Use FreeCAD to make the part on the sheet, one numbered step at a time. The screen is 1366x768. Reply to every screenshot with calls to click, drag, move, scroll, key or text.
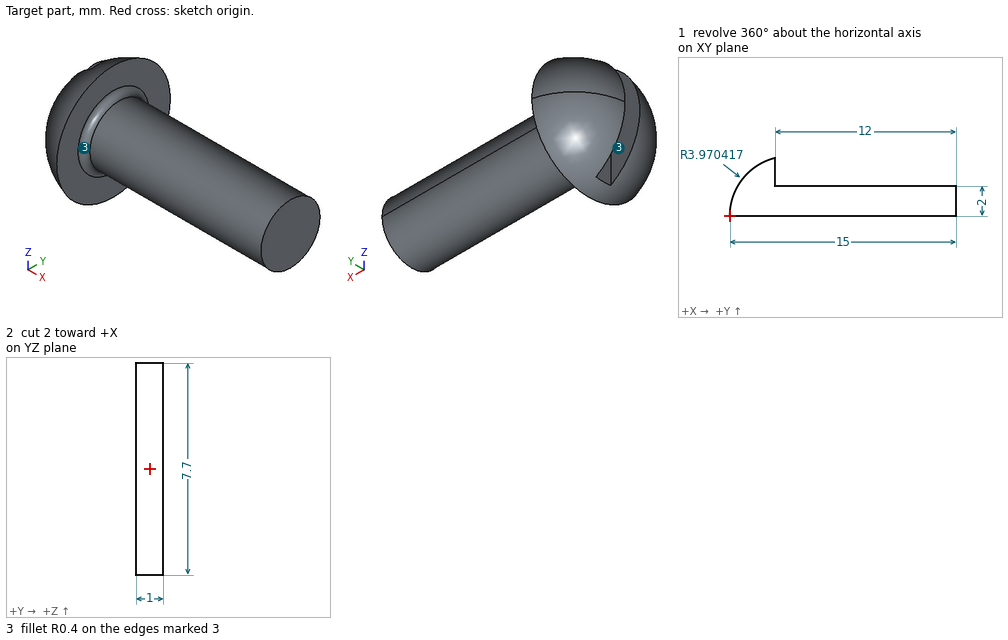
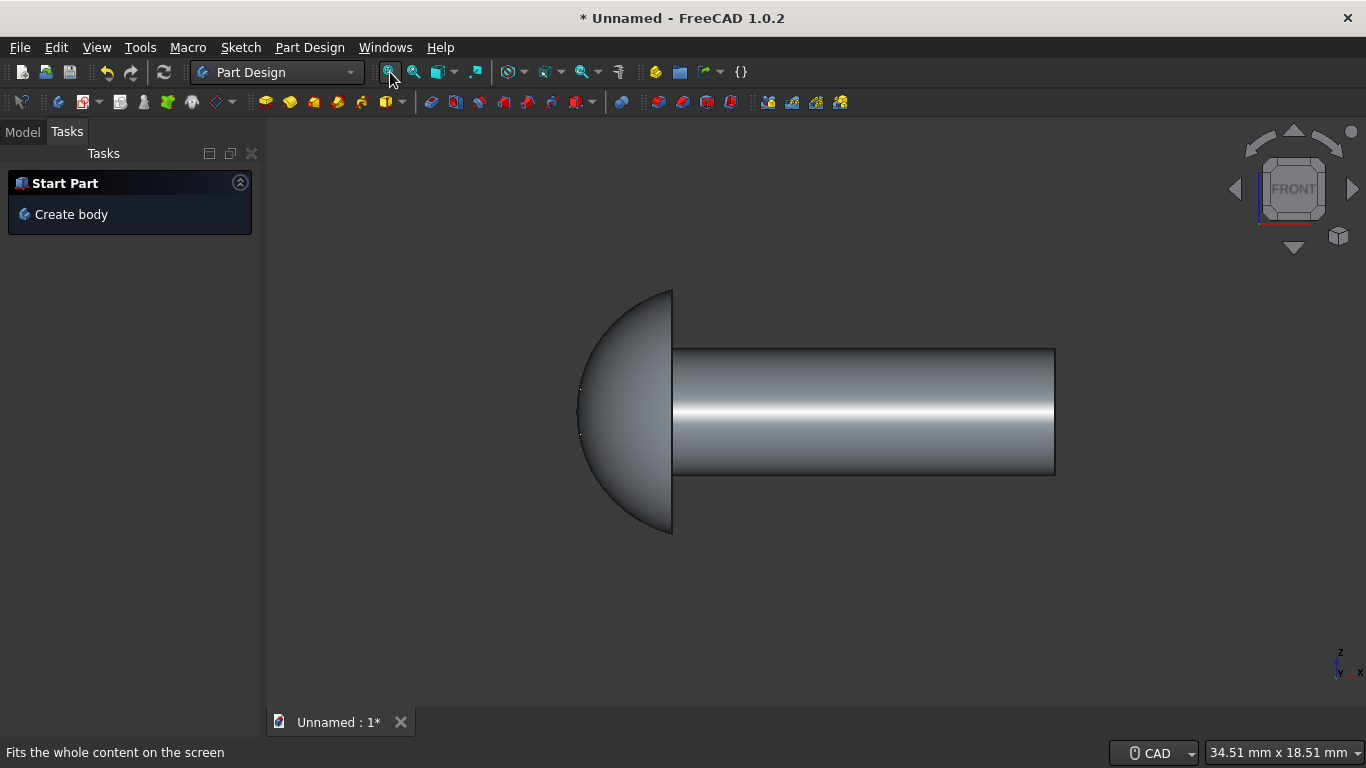
key(v)
key(f)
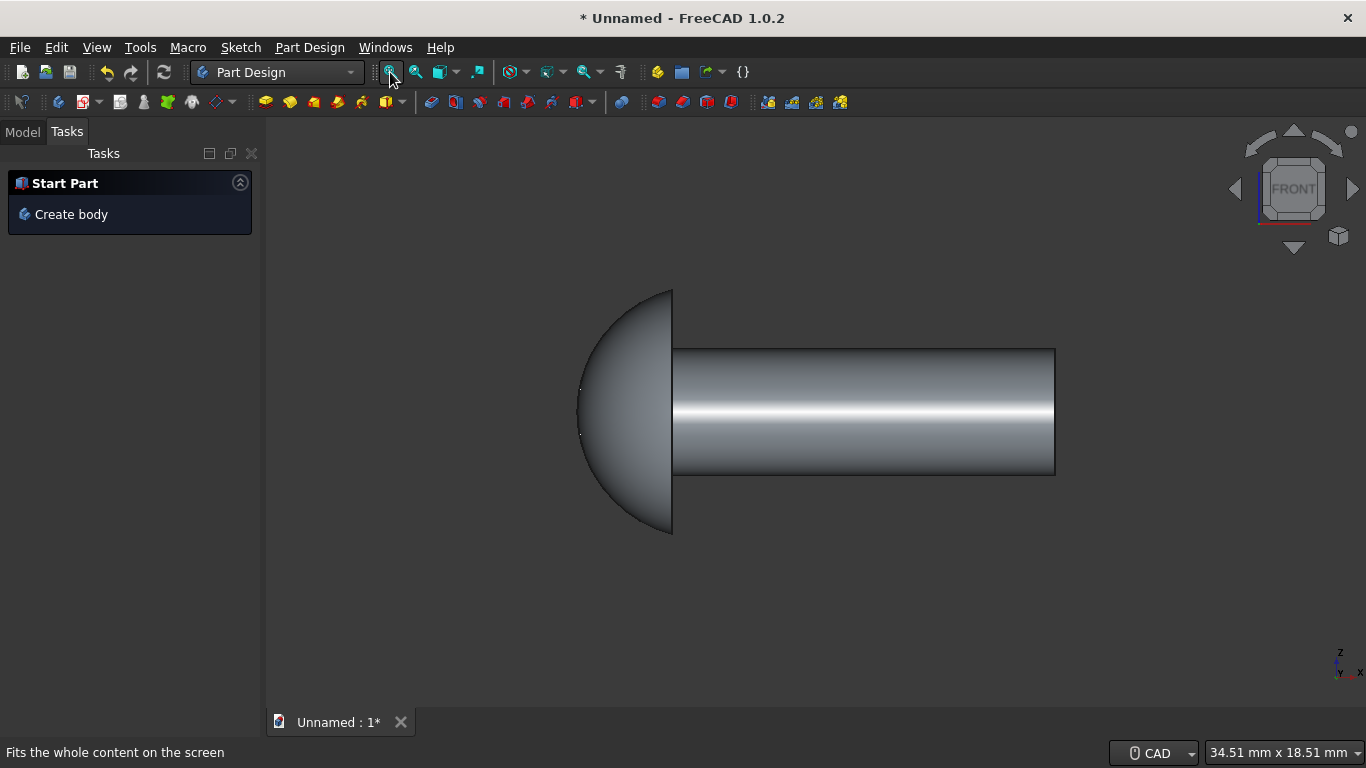
key(3)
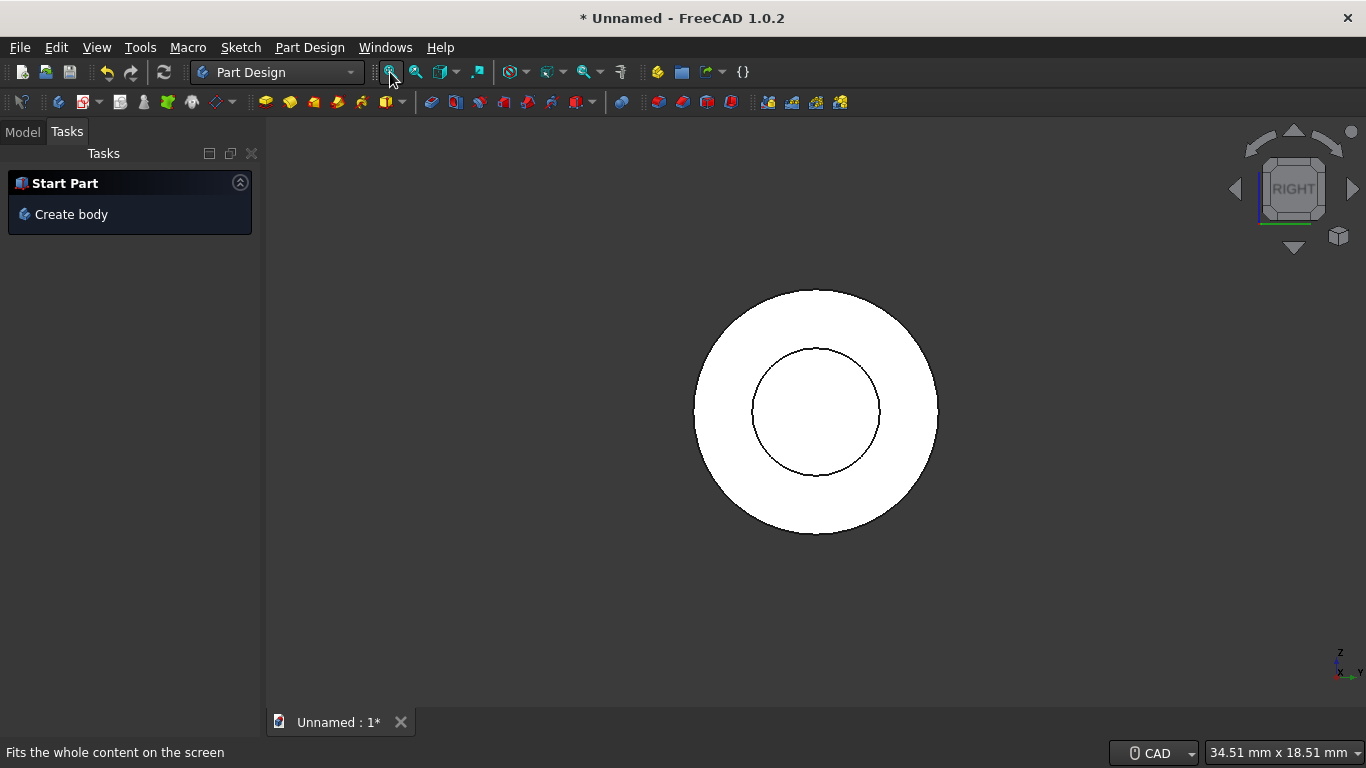
click(392, 72)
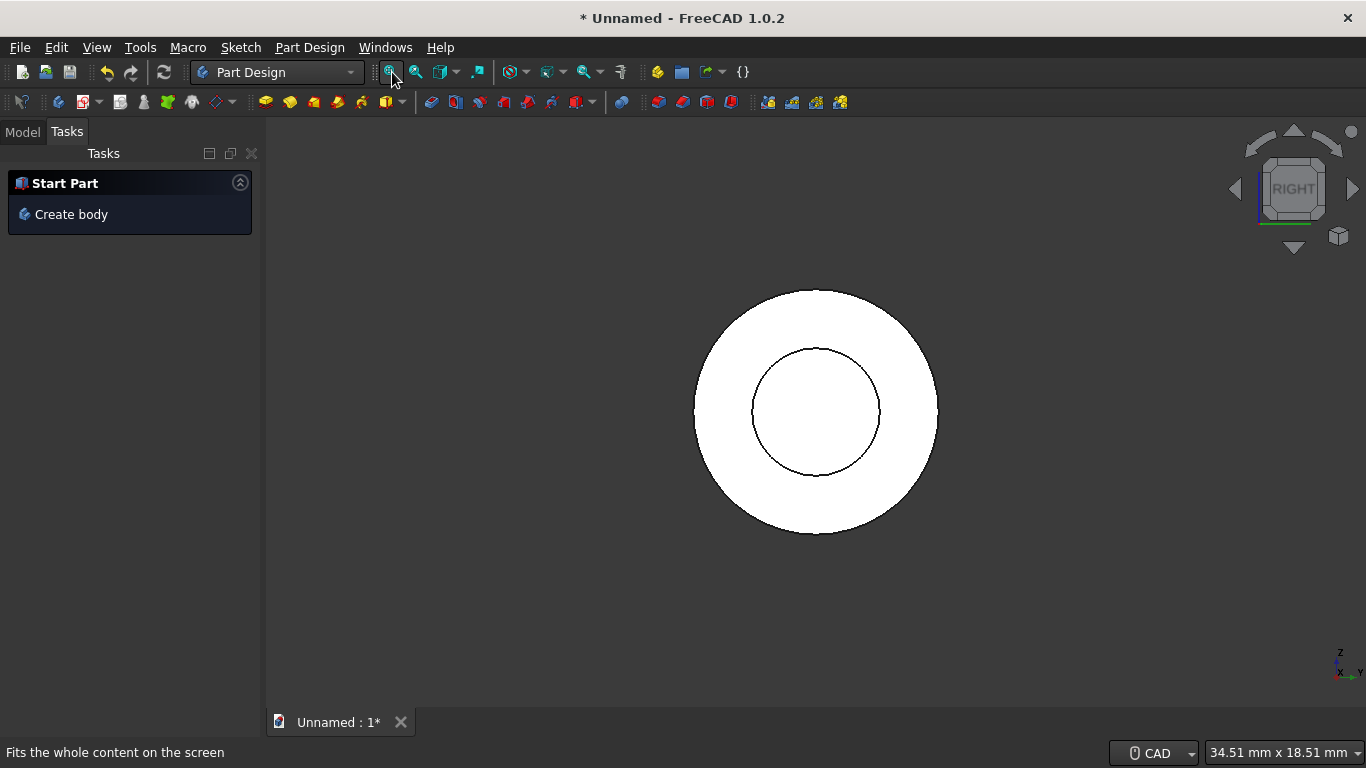
key(5)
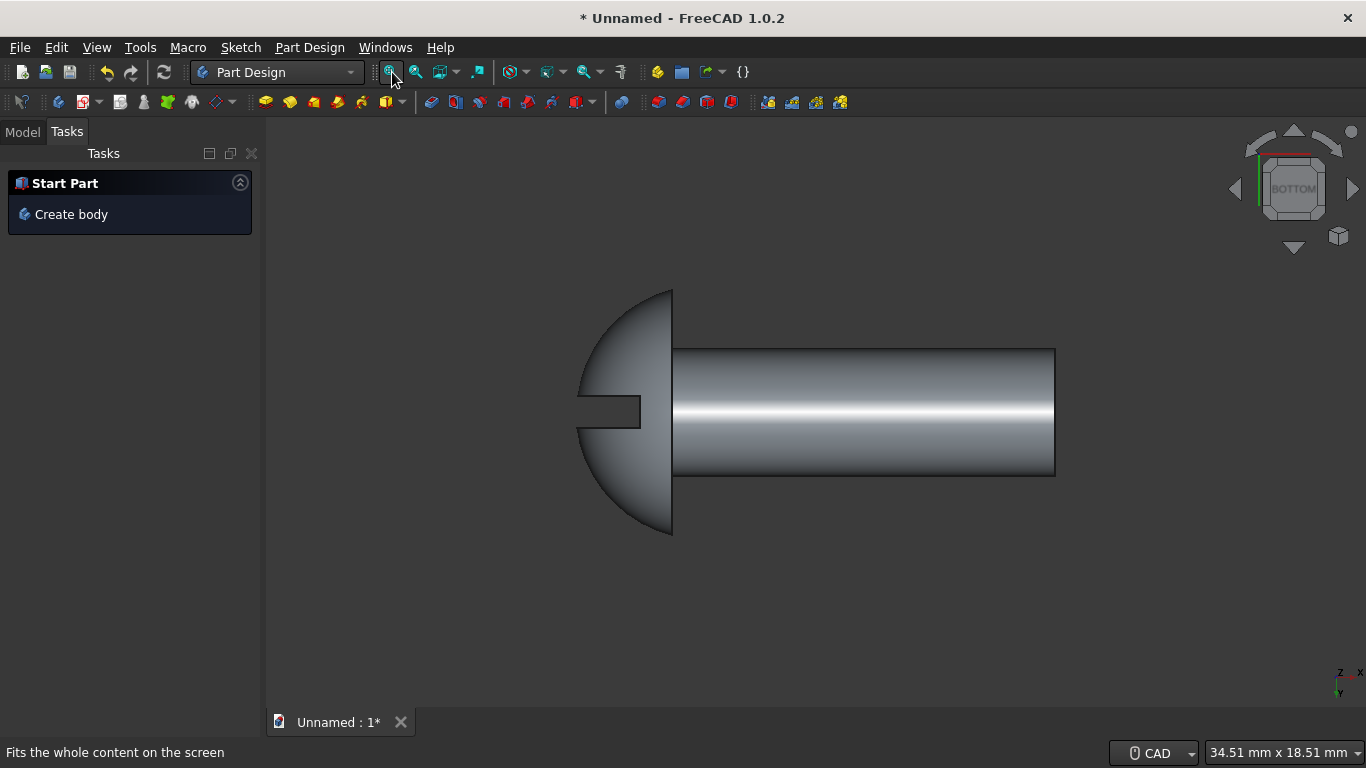
click(392, 72)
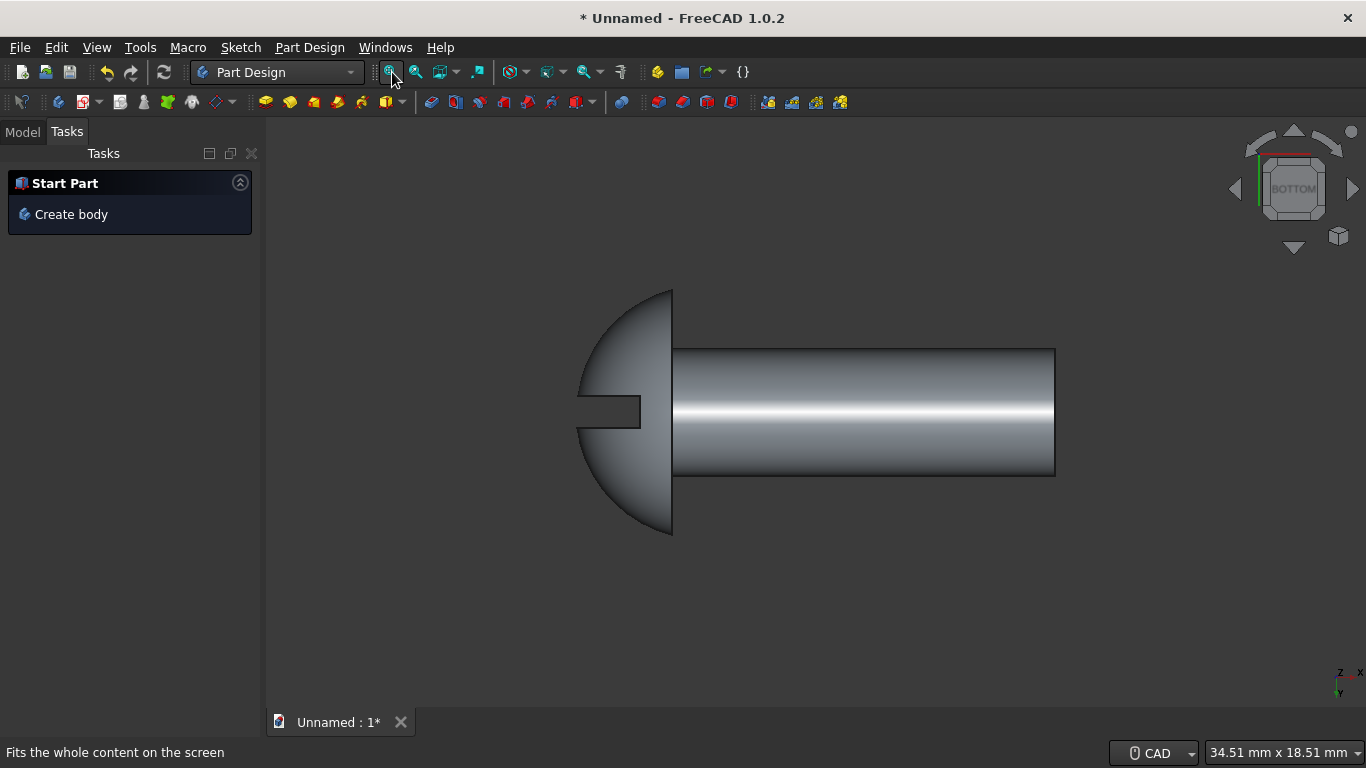
key(4)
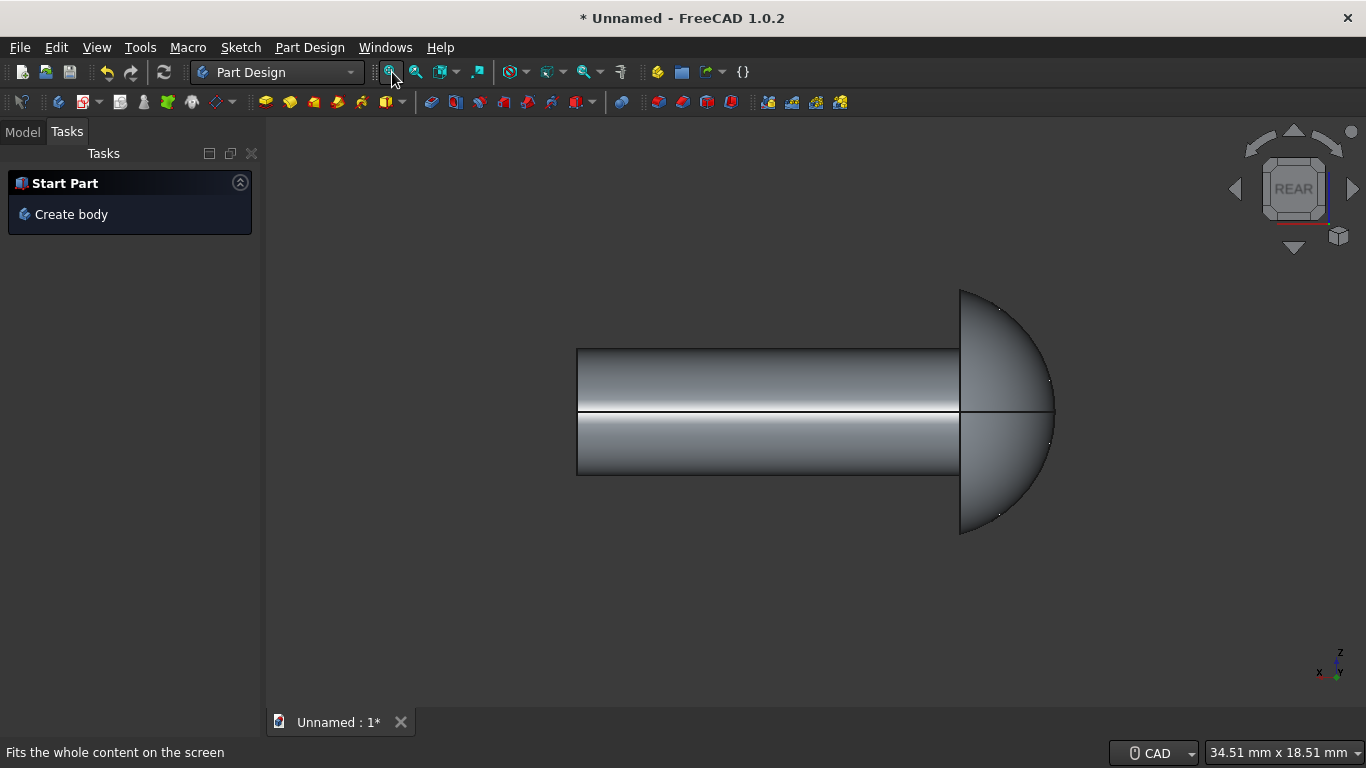
click(392, 72)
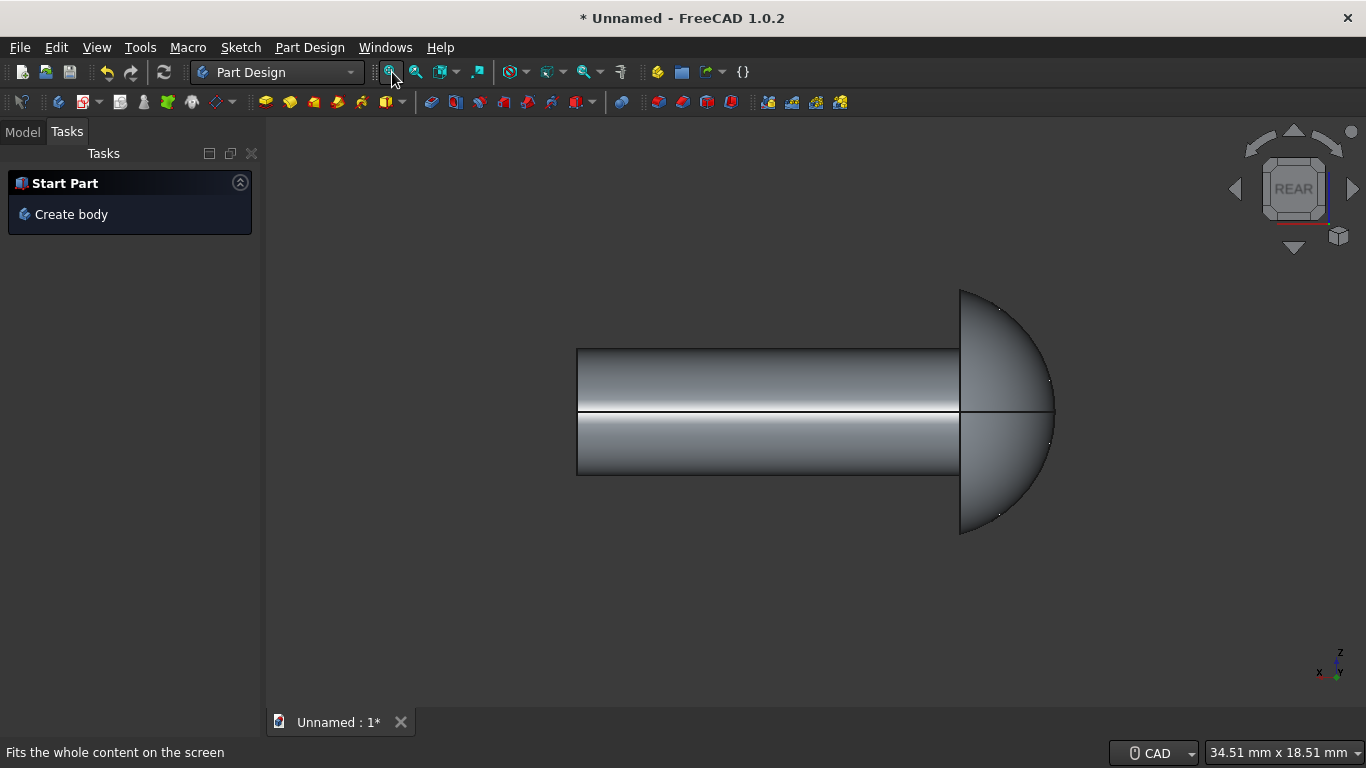
key(6)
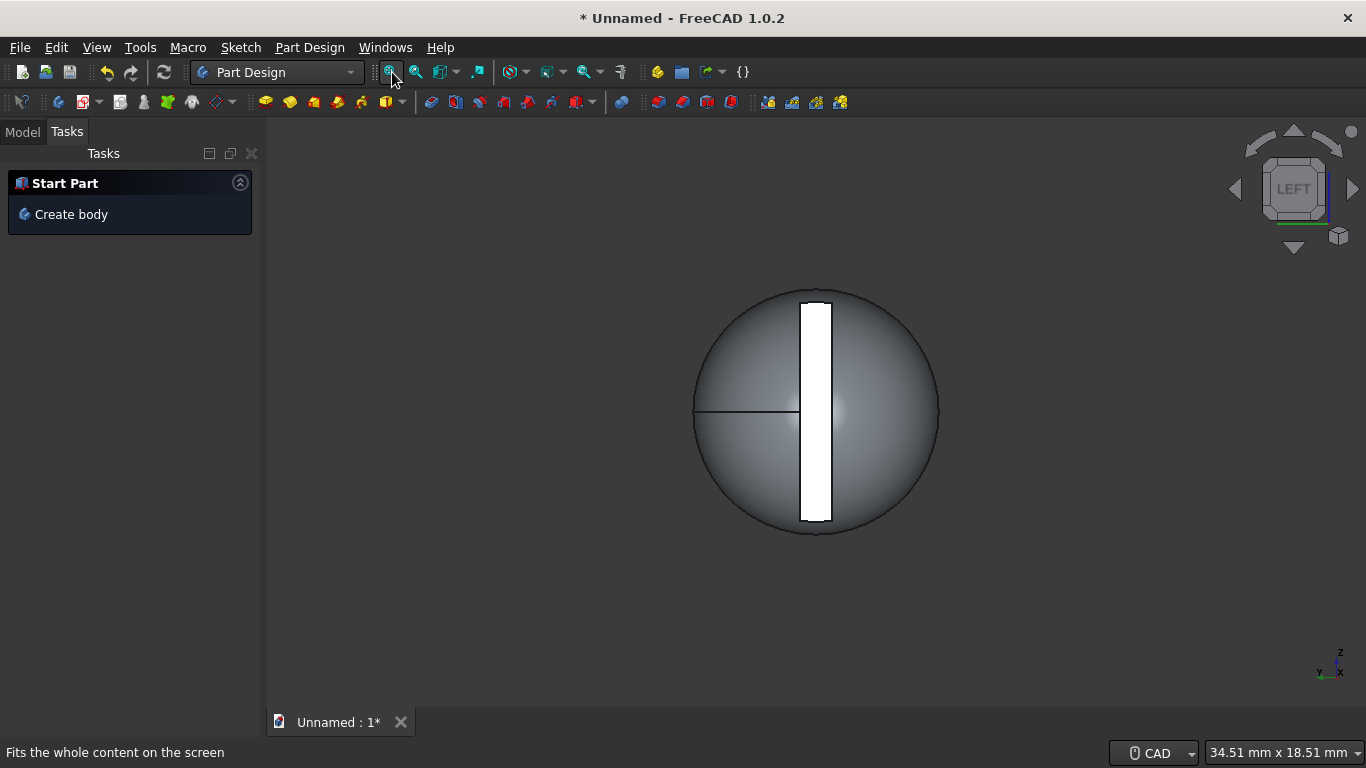
click(392, 72)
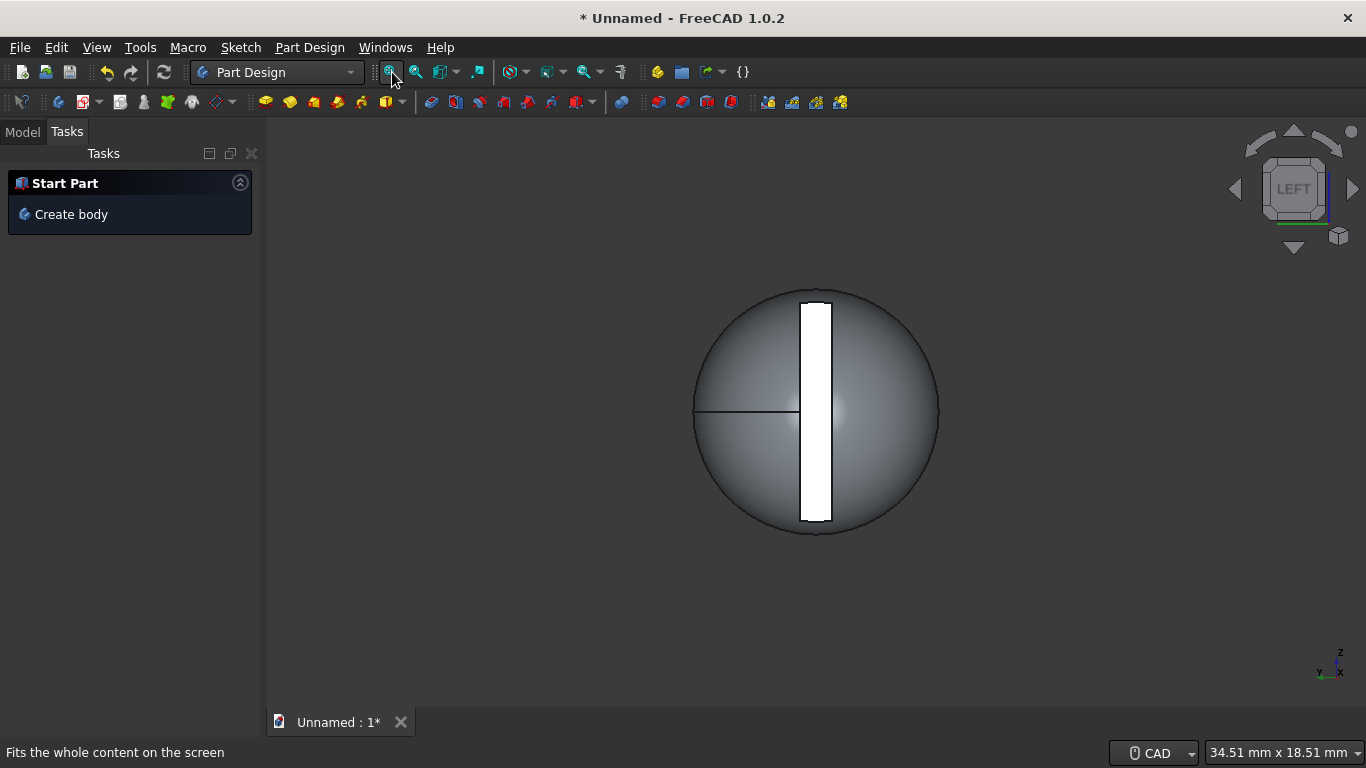
key(v)
key(3)